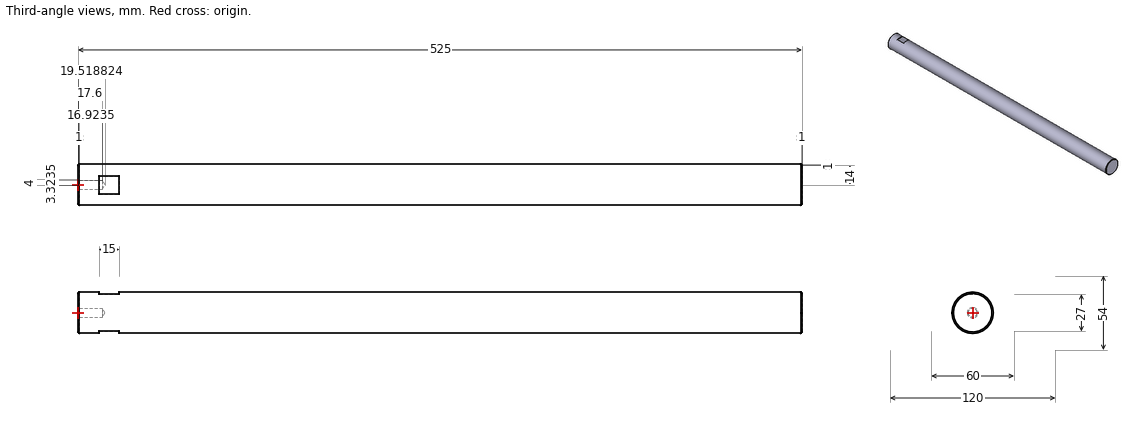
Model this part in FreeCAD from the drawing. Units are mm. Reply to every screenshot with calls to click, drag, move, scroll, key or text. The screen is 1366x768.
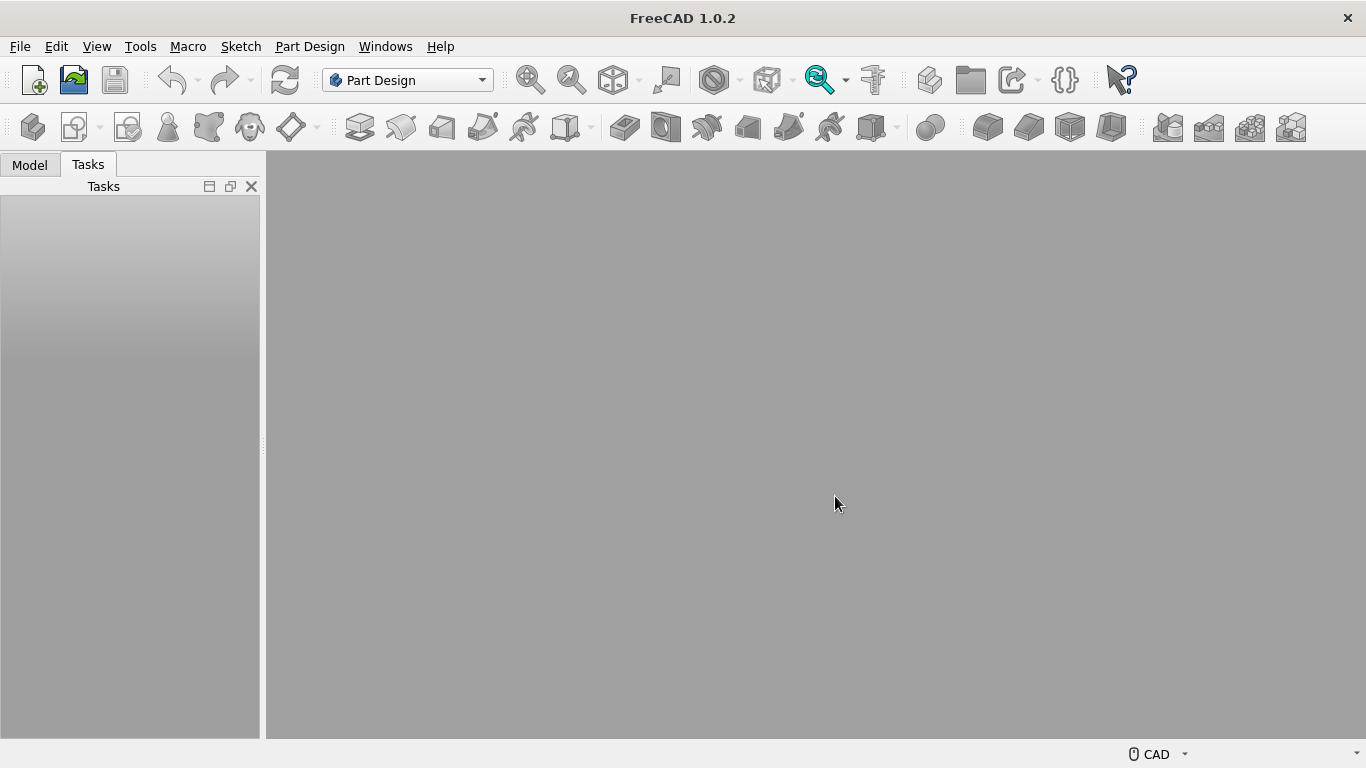
click(33, 80)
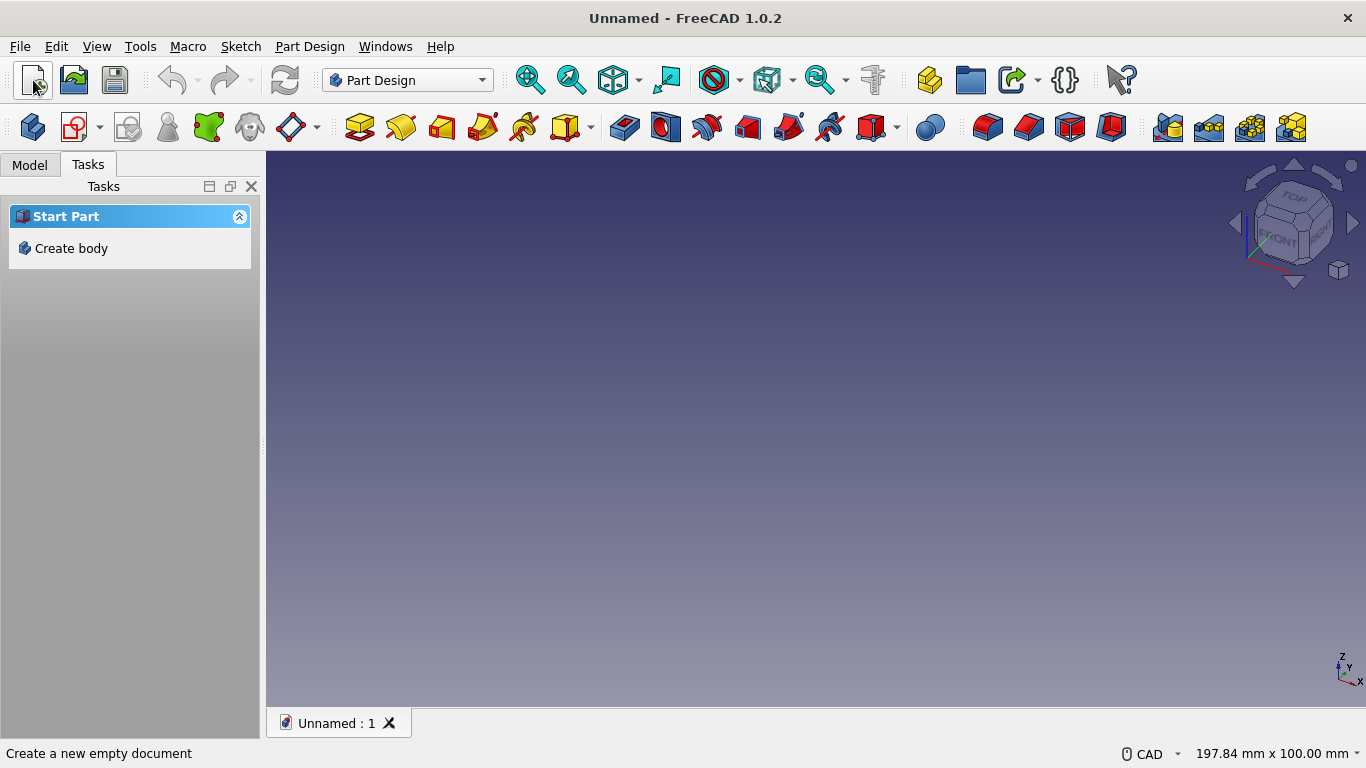
click(74, 128)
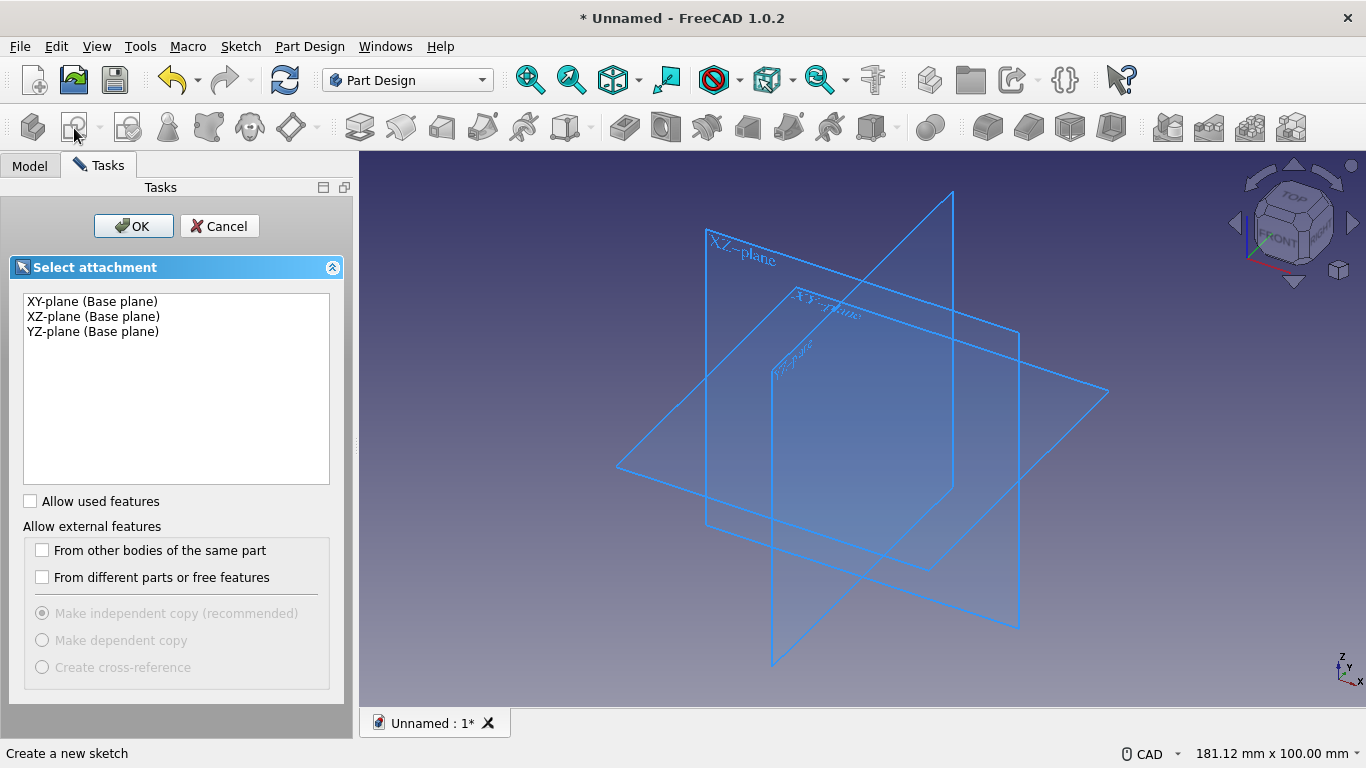
click(84, 302)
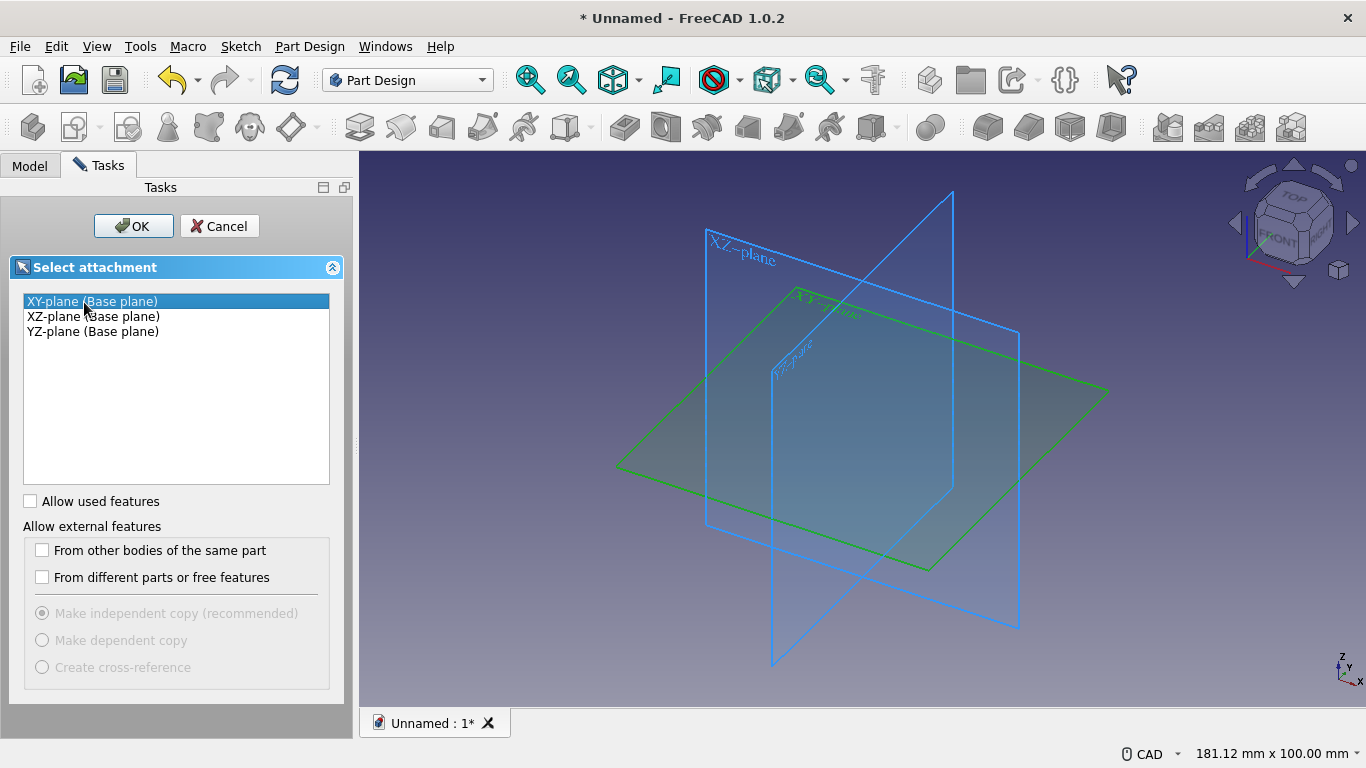
click(134, 226)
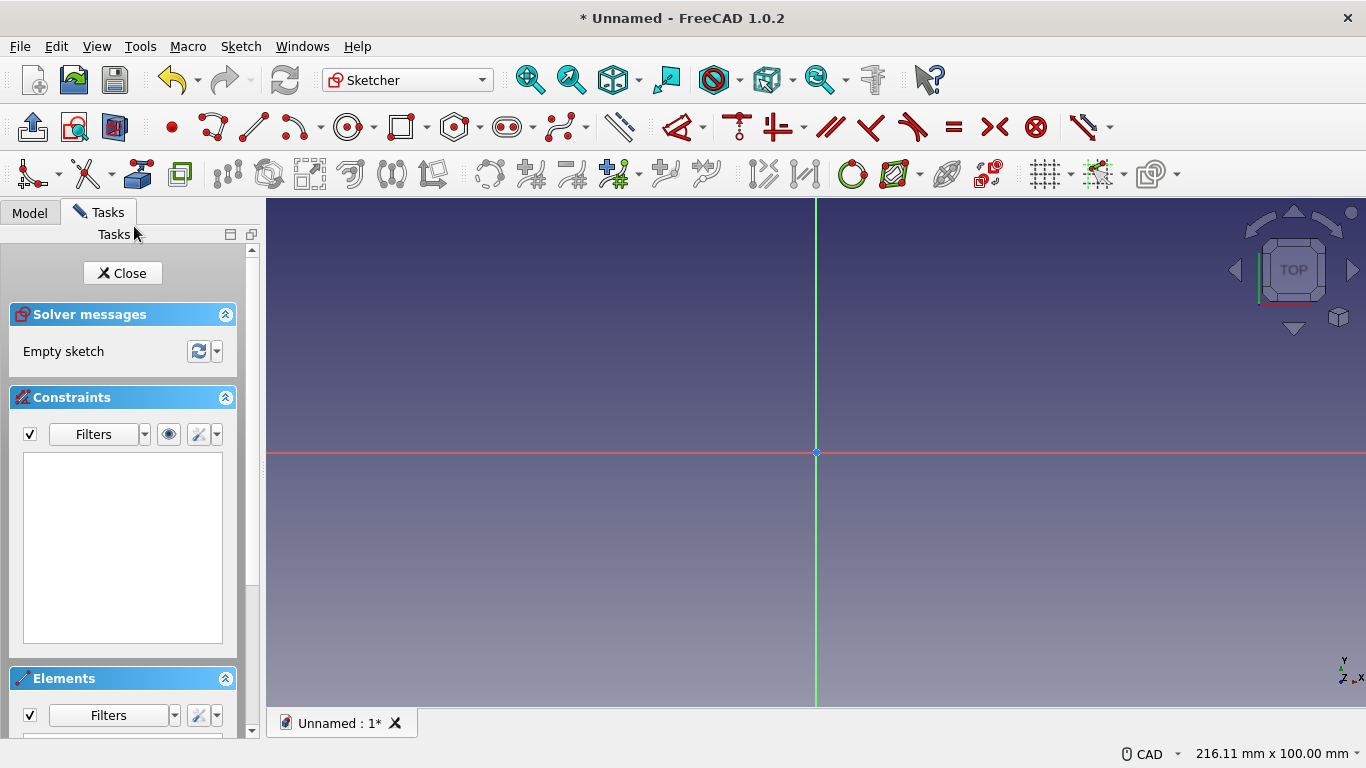
scroll(294, 465, down, 7)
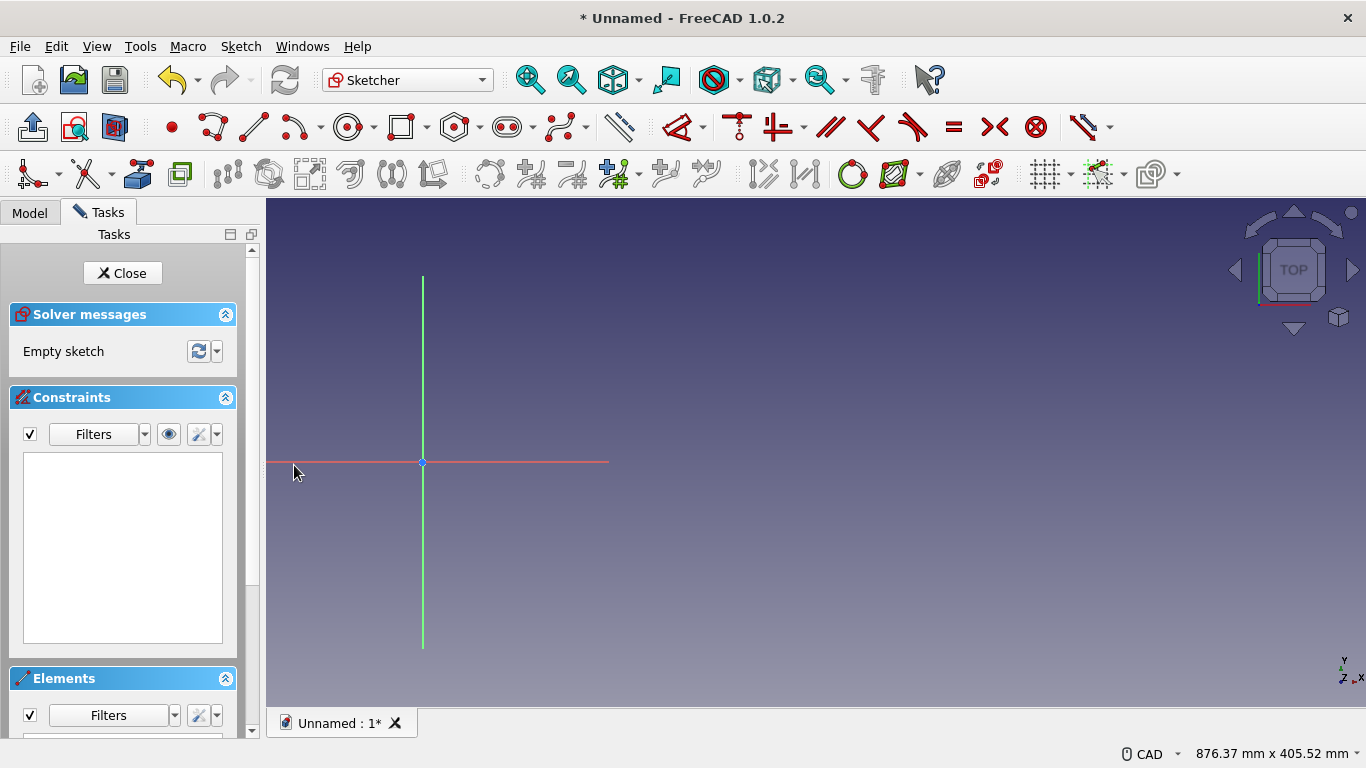
click(213, 128)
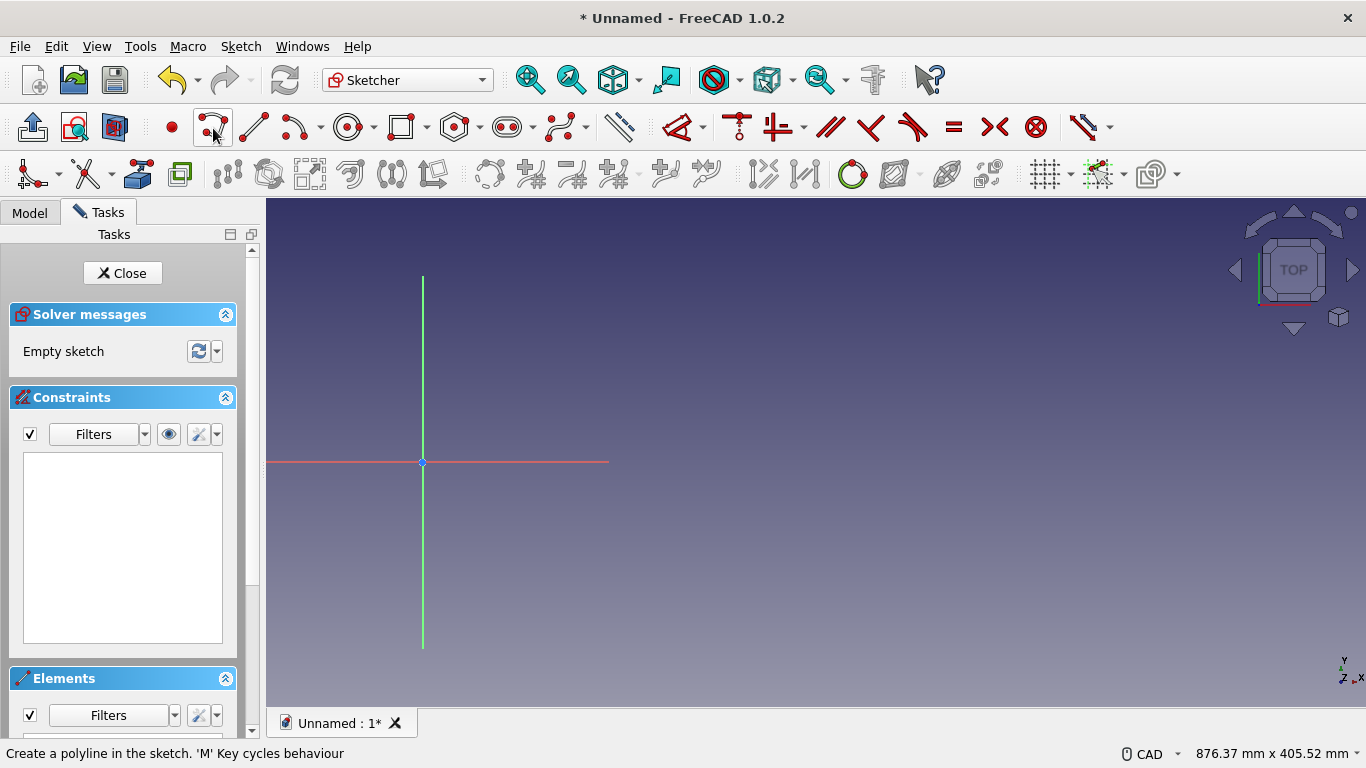
click(423, 462)
click(1082, 453)
click(1082, 445)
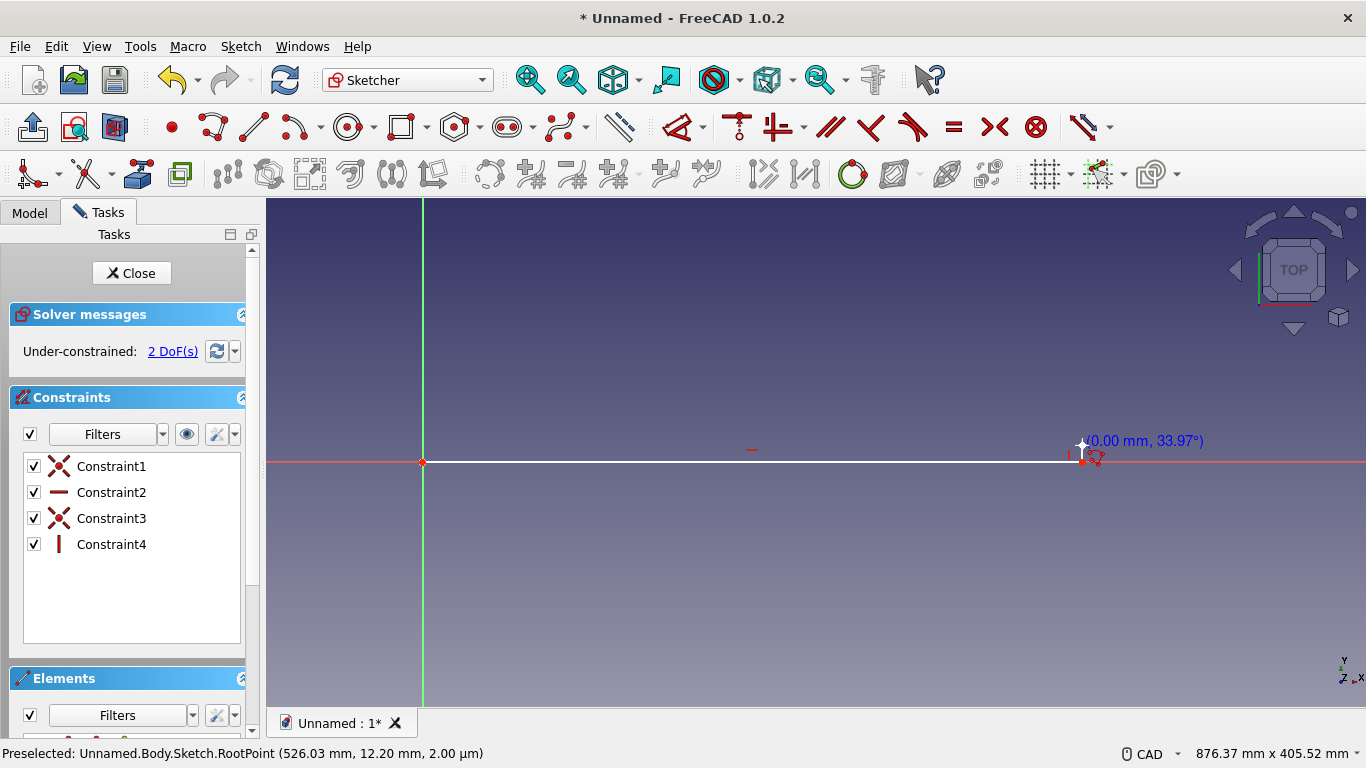
scroll(1080, 443, up, 11)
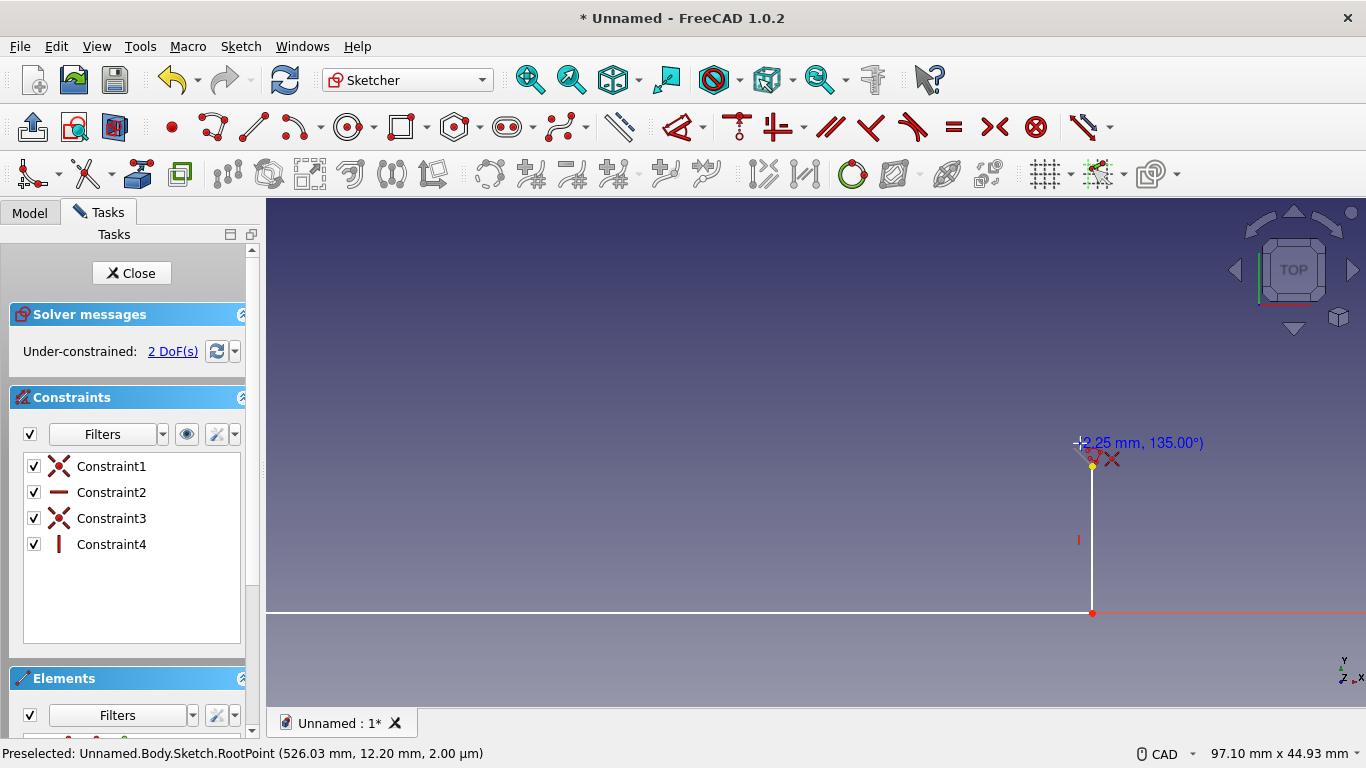
click(1078, 444)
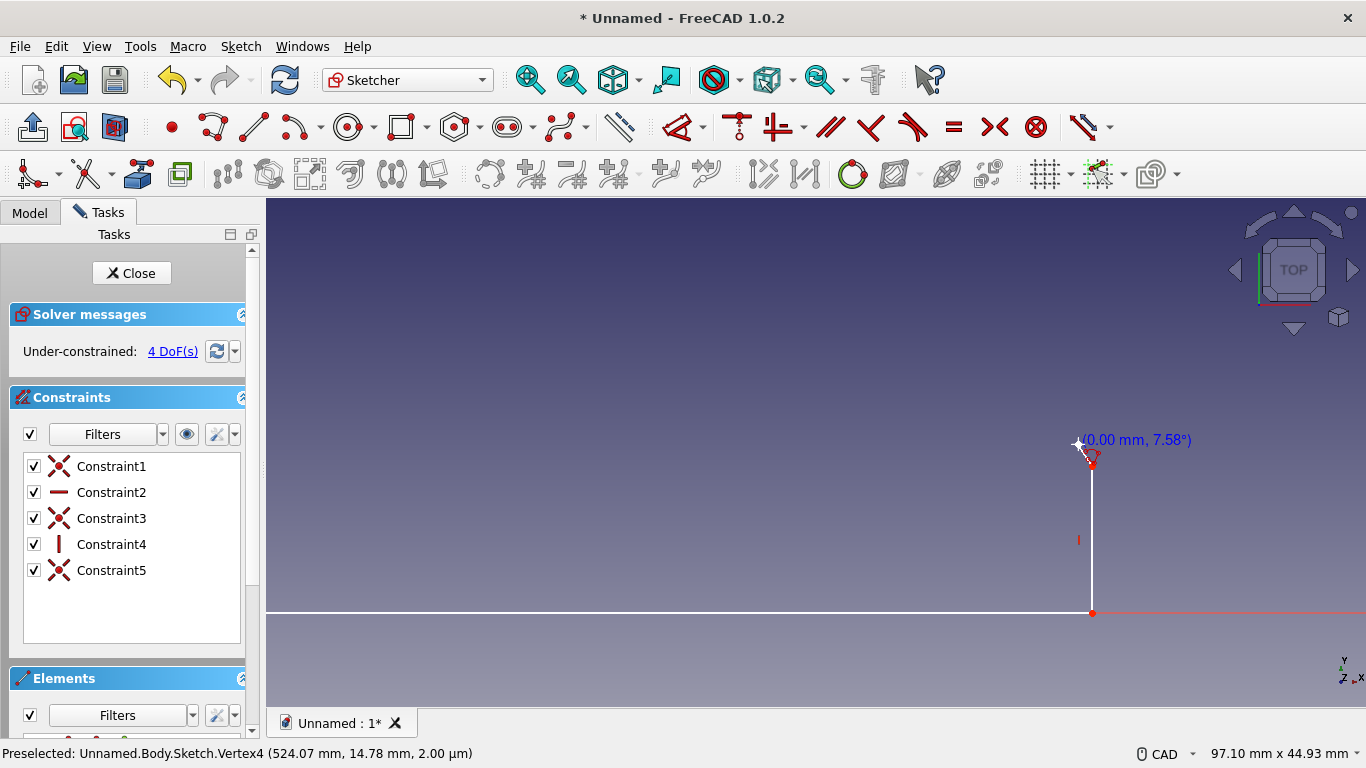
scroll(1075, 443, down, 11)